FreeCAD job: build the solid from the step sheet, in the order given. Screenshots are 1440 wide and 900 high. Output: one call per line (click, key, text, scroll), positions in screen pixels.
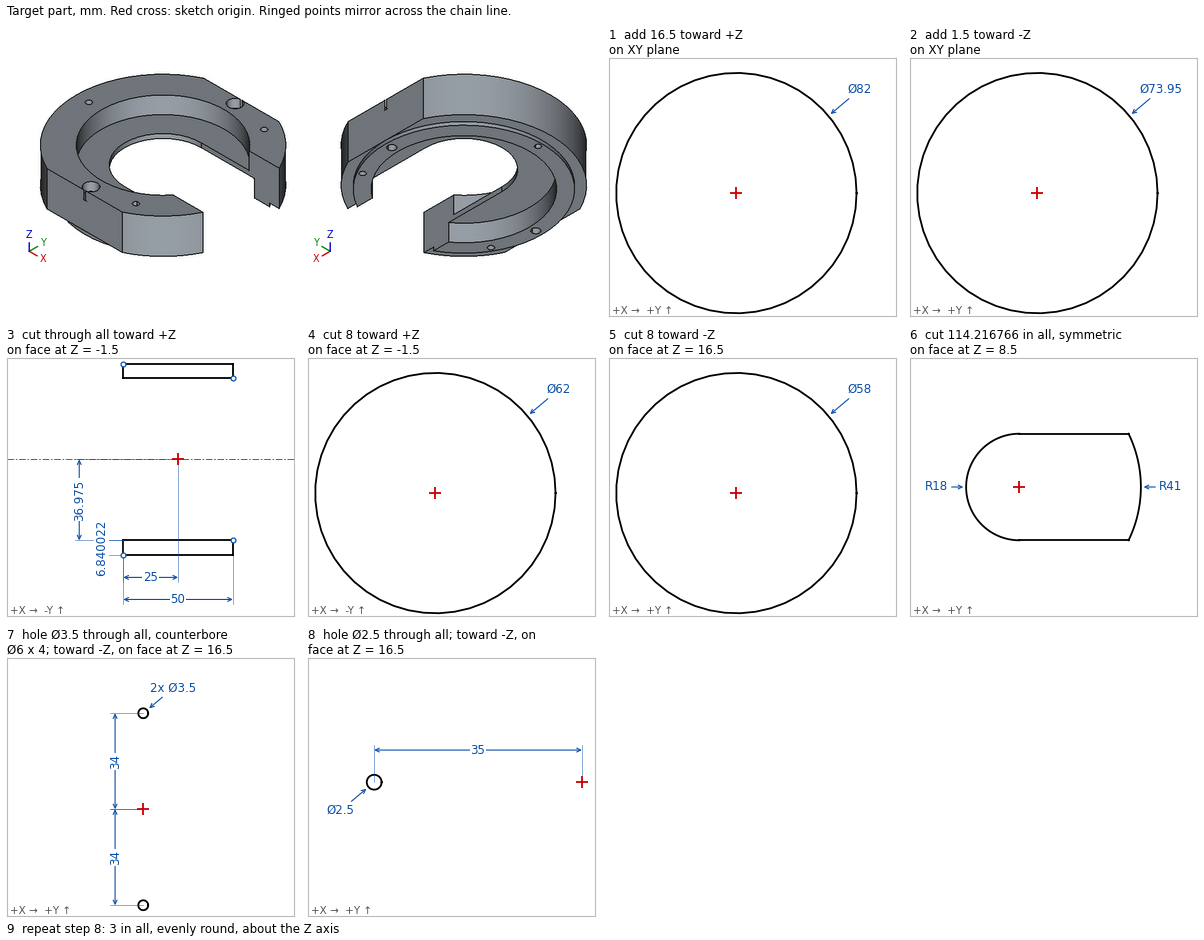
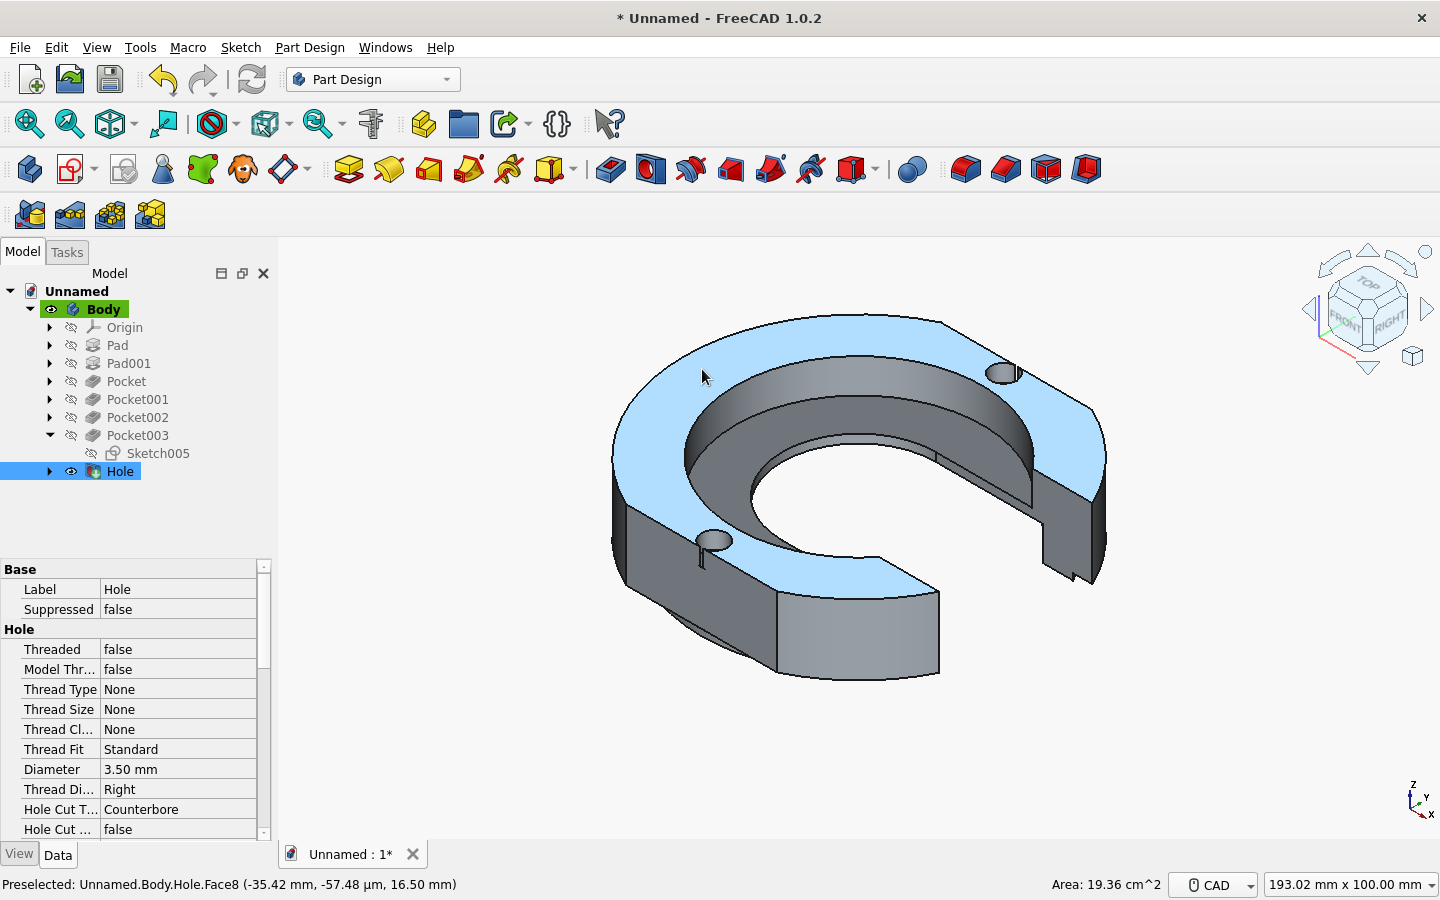
click(70, 170)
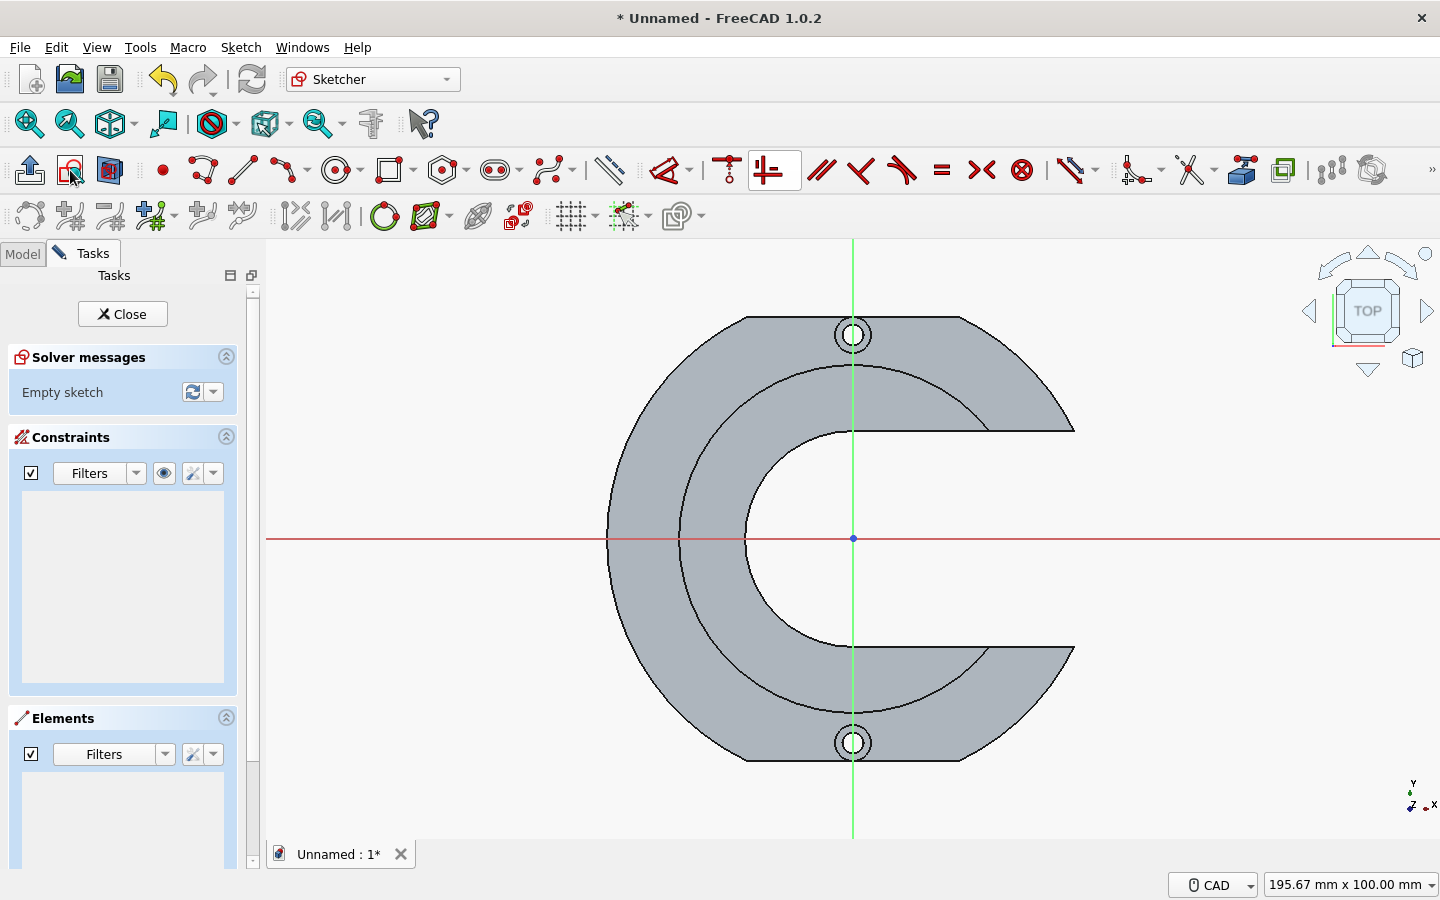
scroll(636, 539, up, 15)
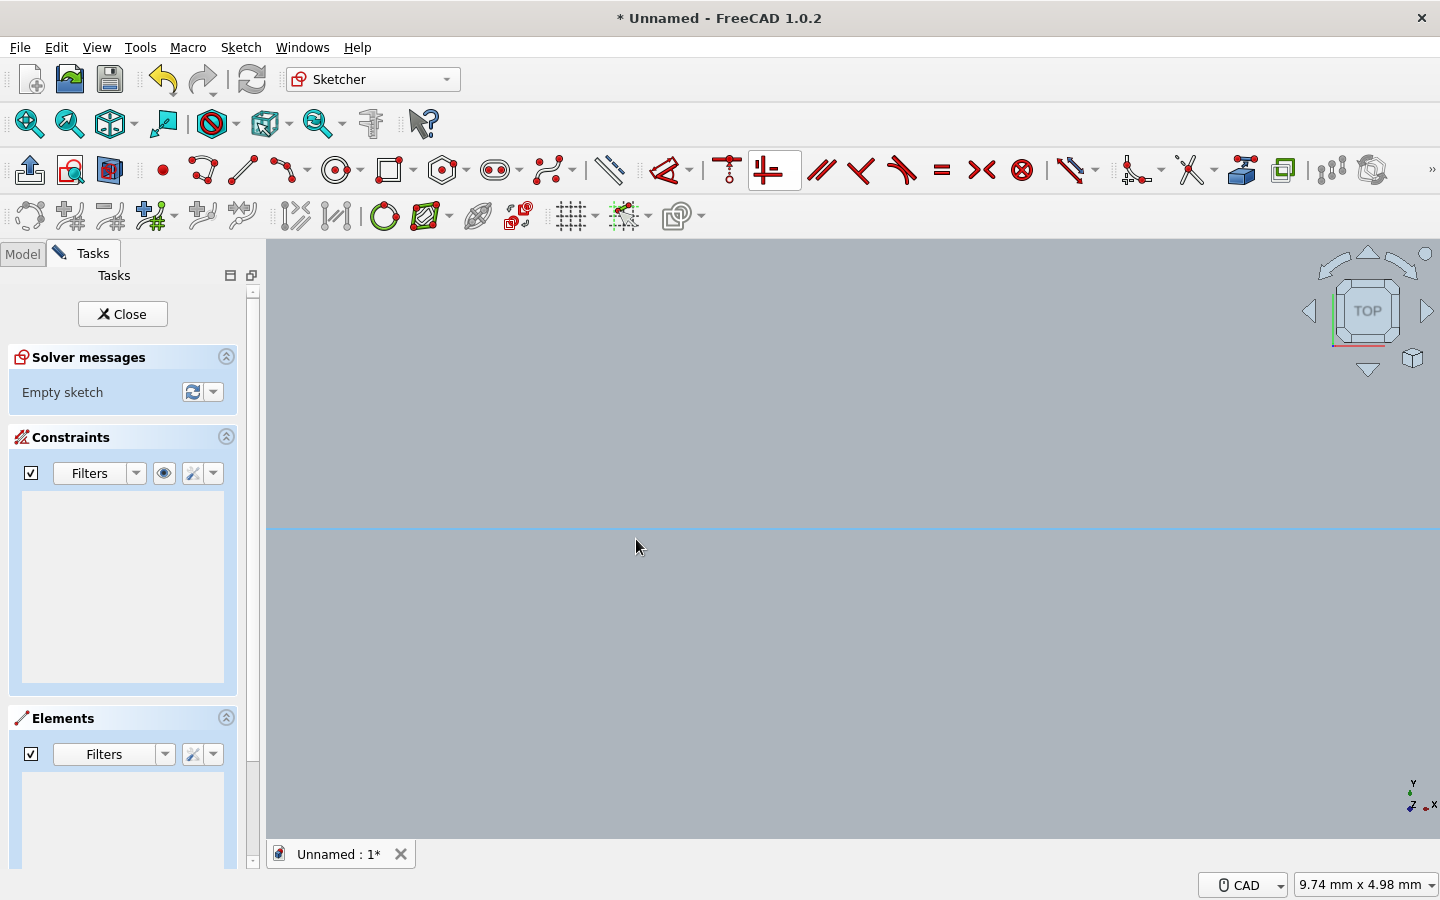
key(g)
key(c)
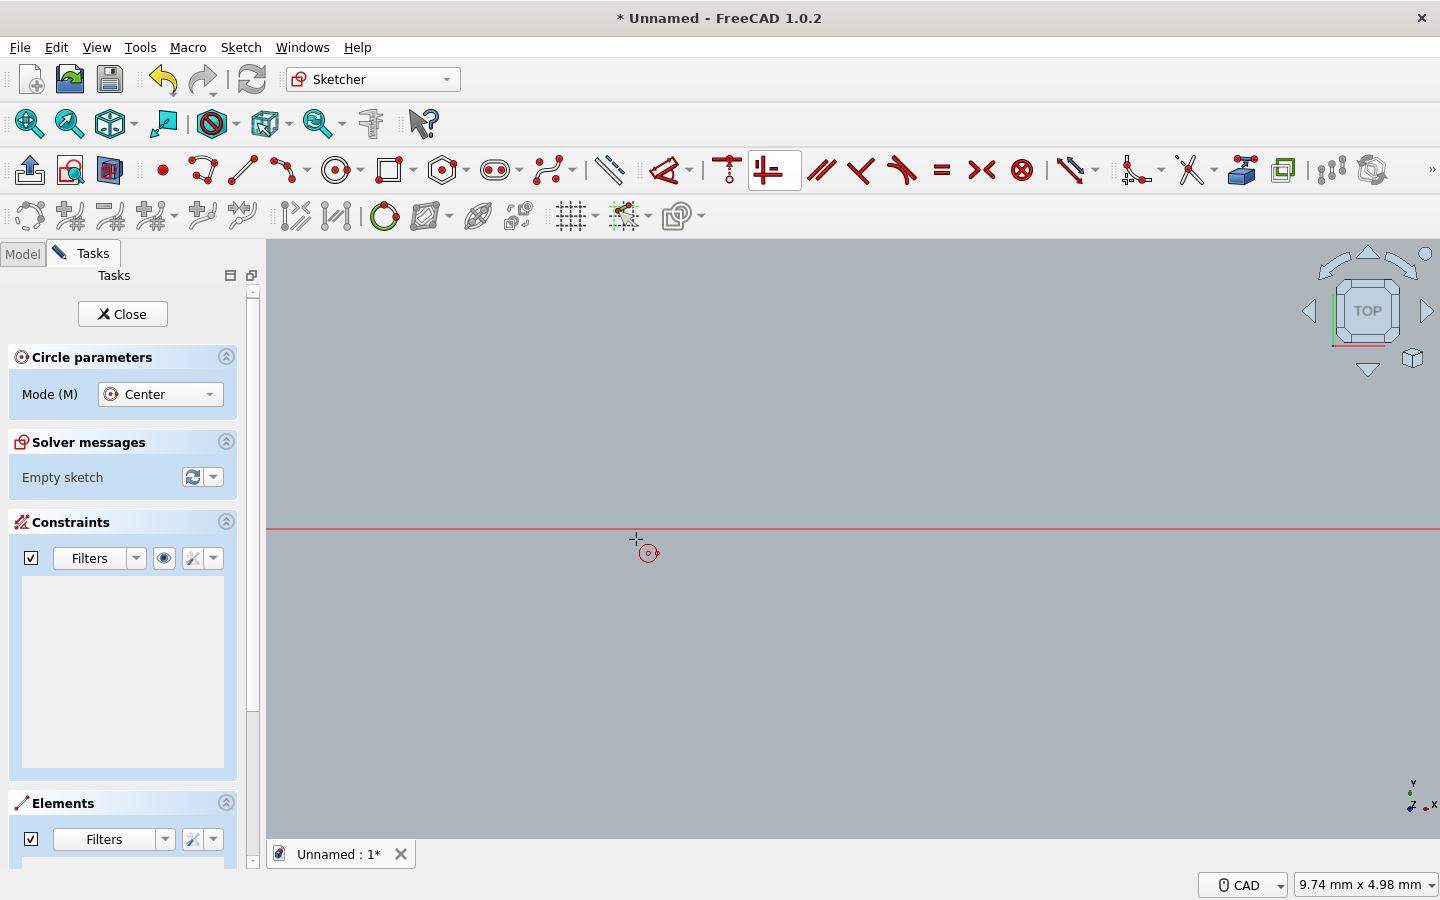
click(771, 529)
click(877, 423)
key(Escape)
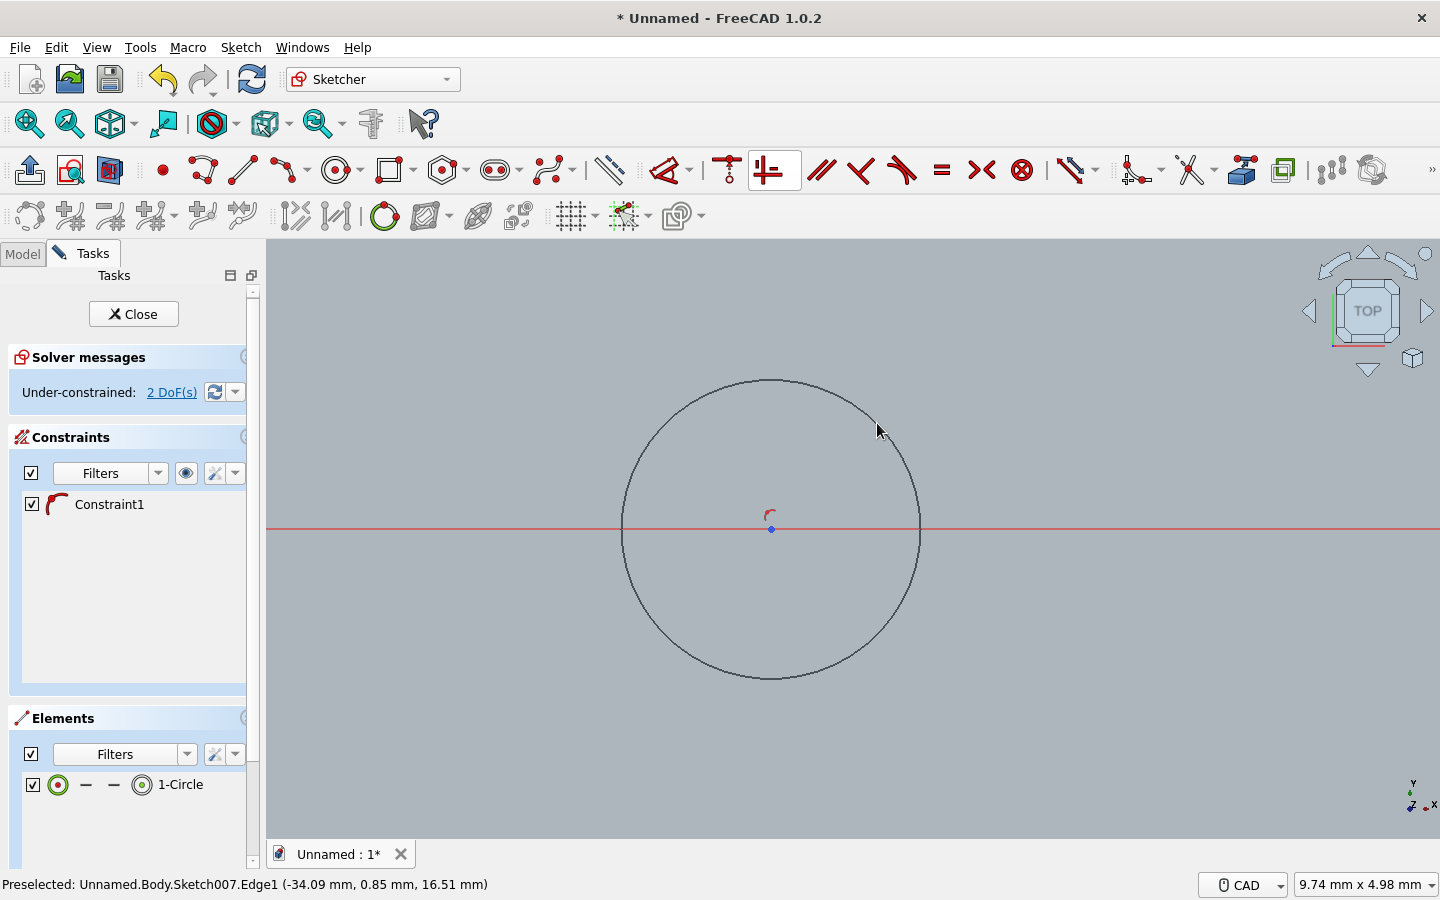
key(d)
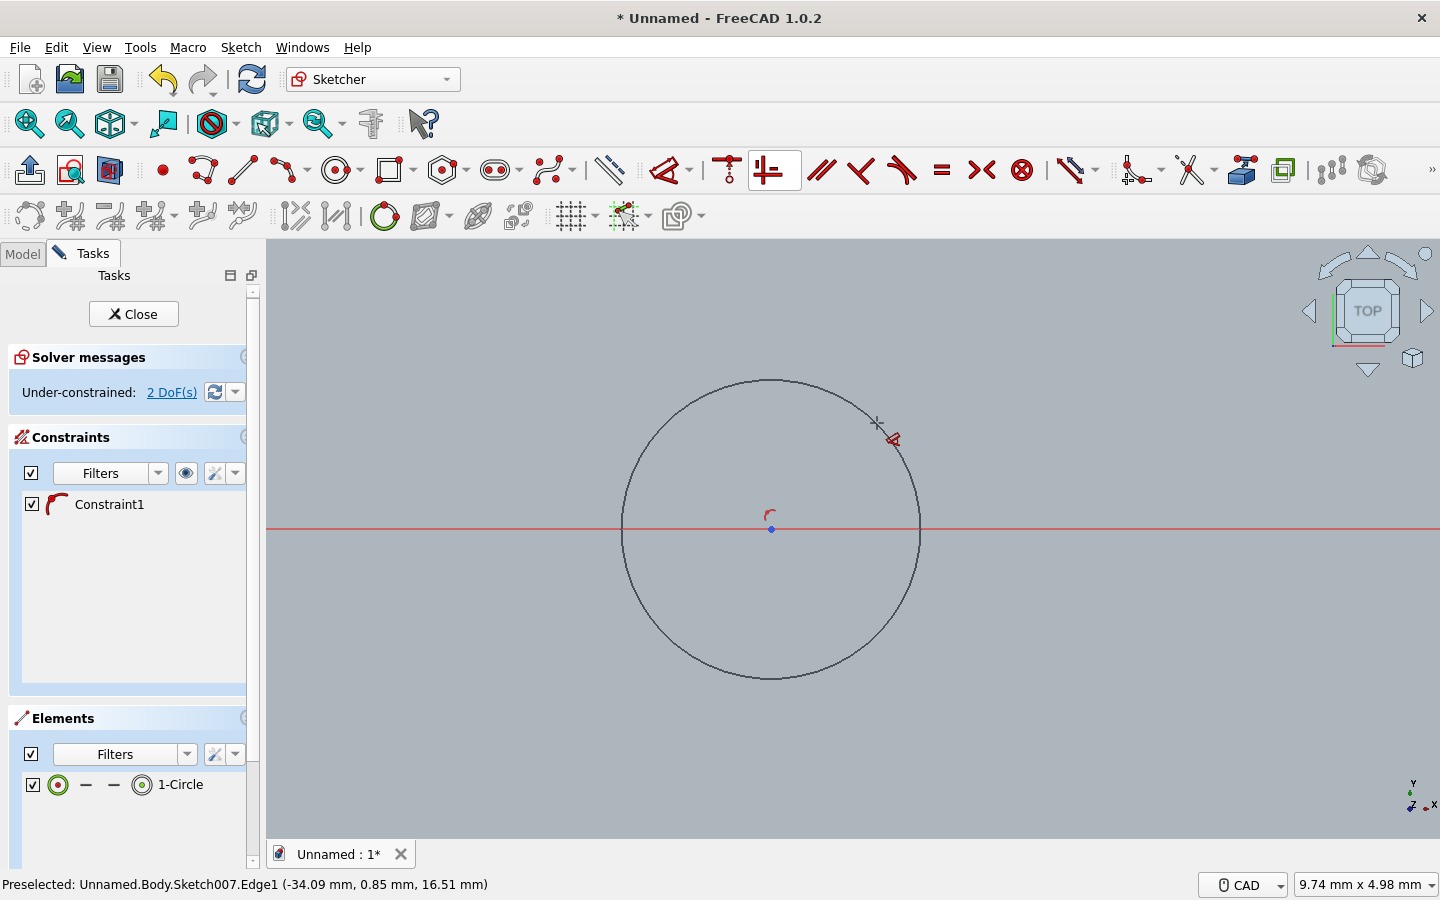
click(876, 423)
click(898, 400)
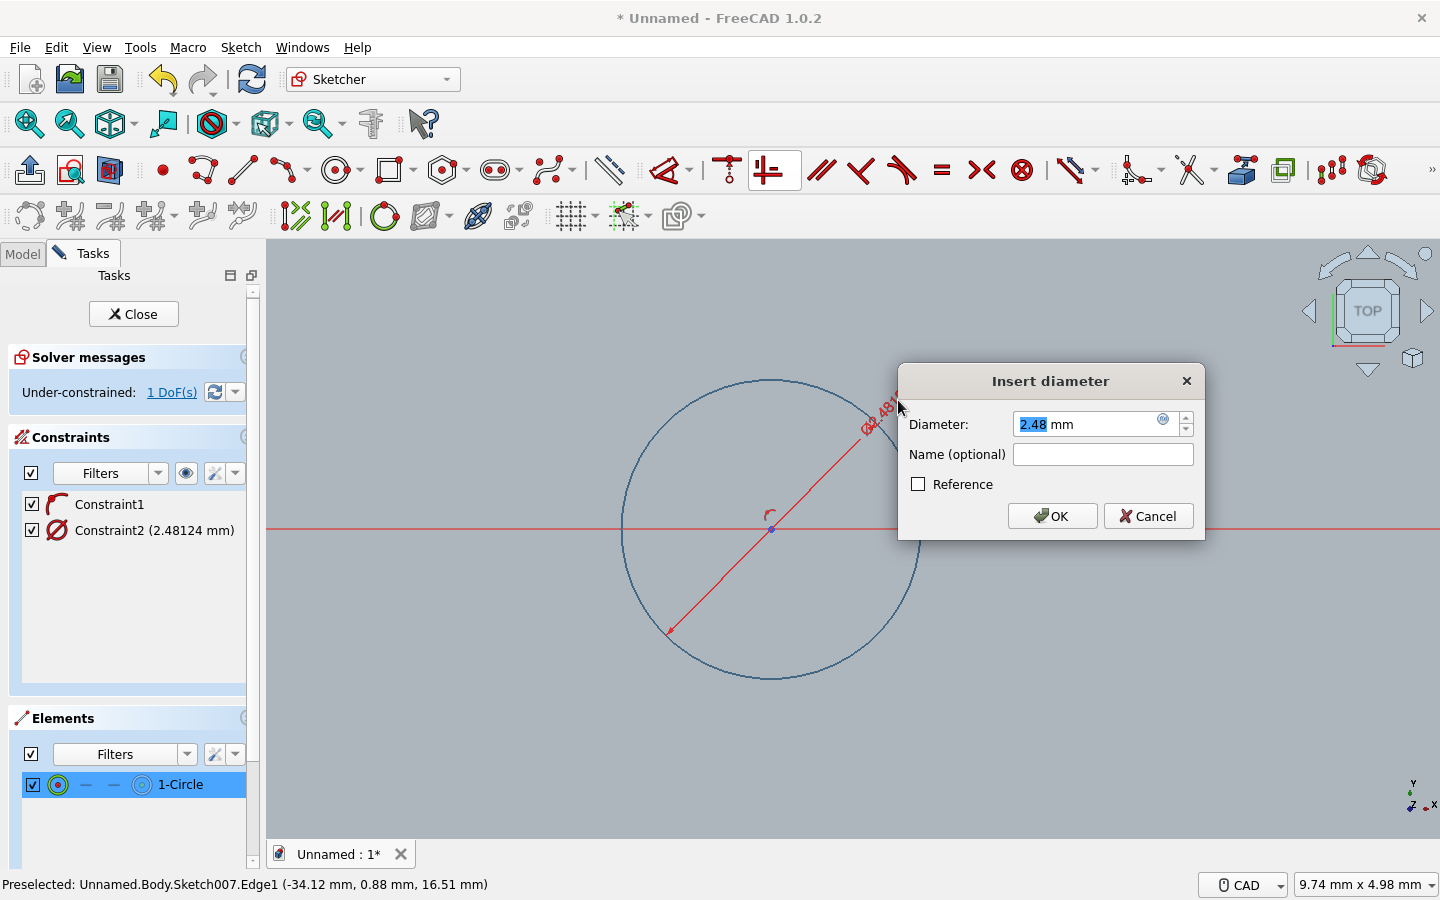
text(2.5)
key(Return)